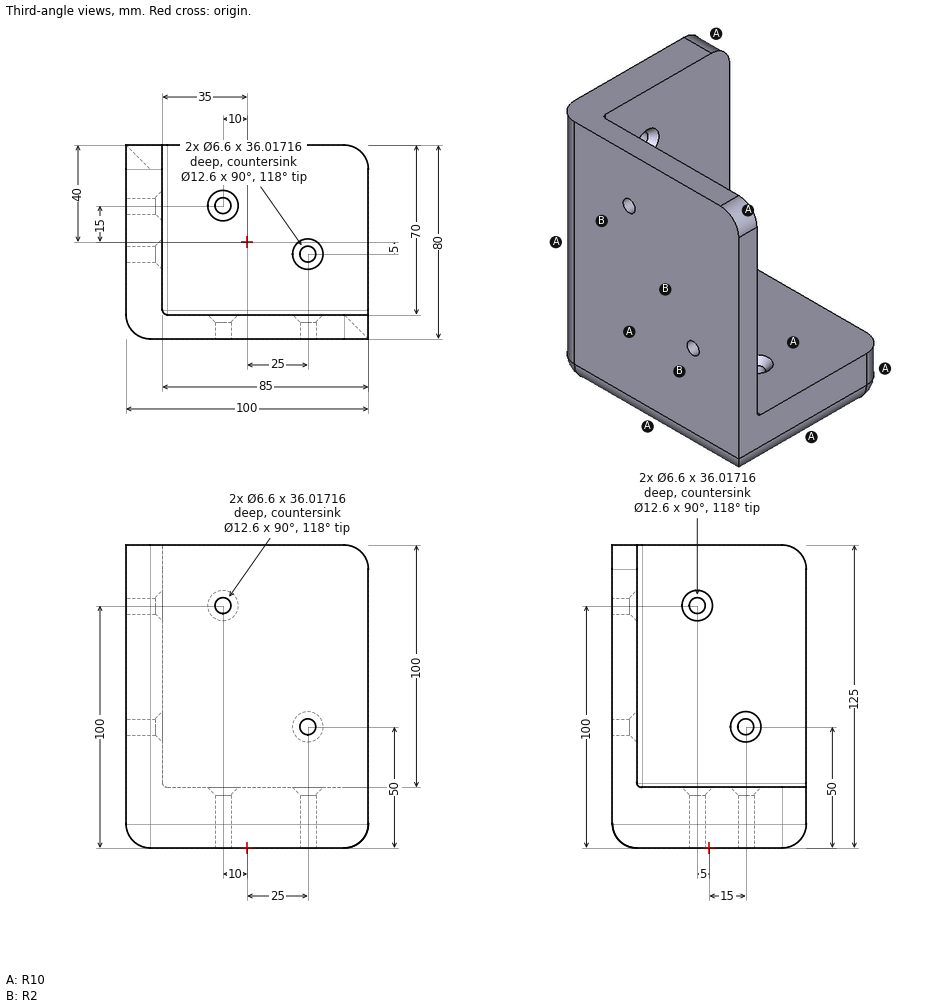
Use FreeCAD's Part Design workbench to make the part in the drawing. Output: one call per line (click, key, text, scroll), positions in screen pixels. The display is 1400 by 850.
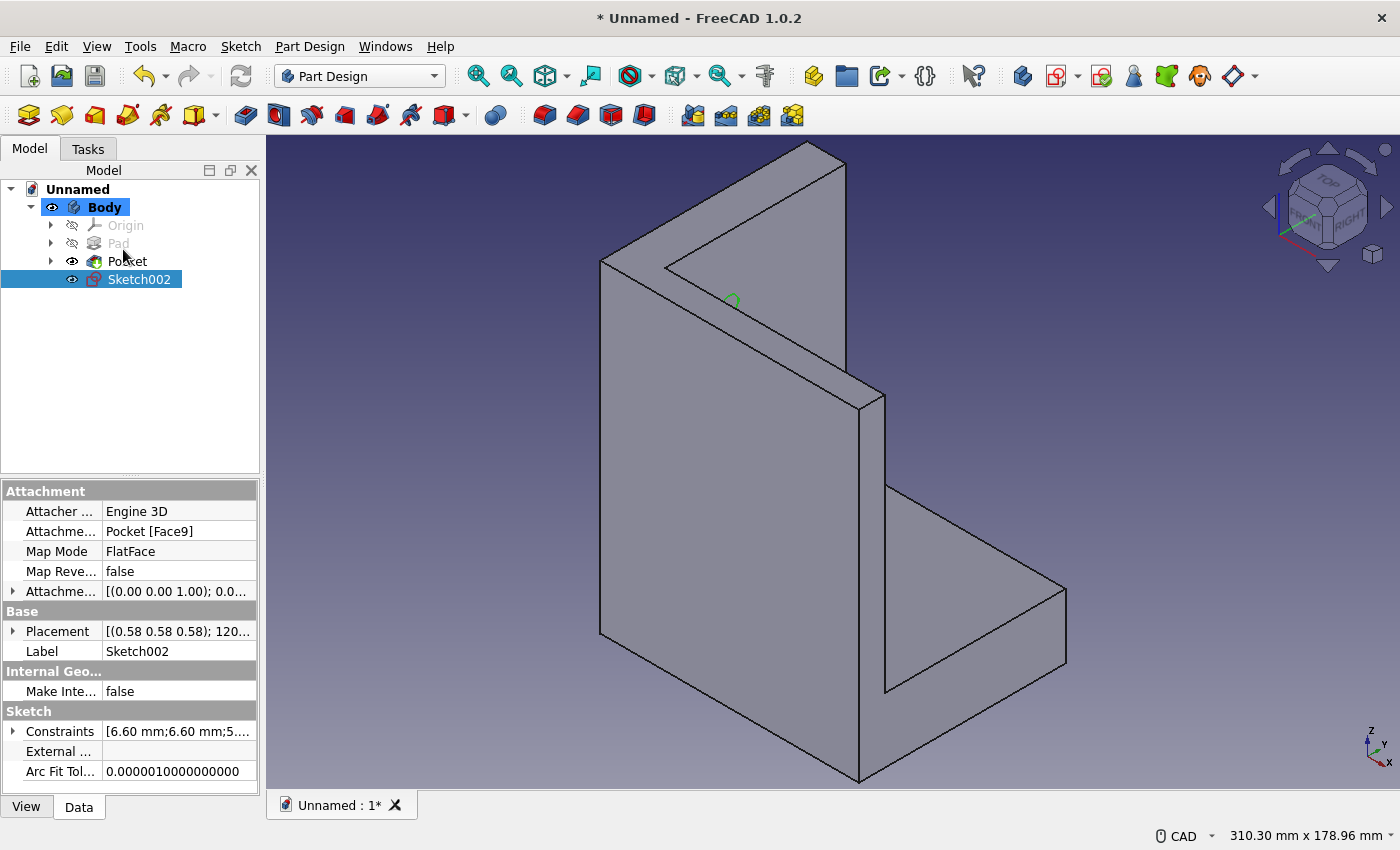
click(279, 116)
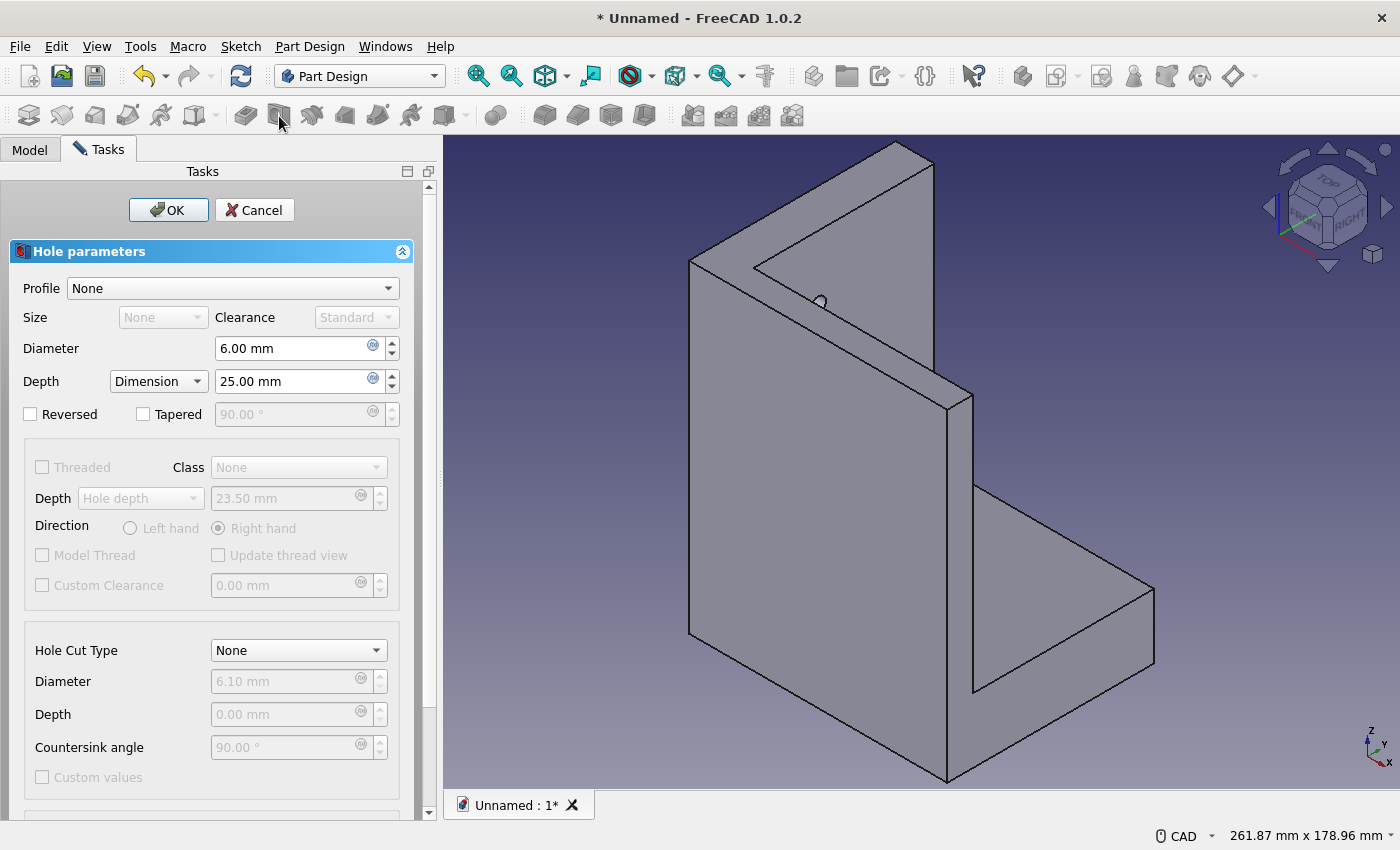
triple_click(300, 348)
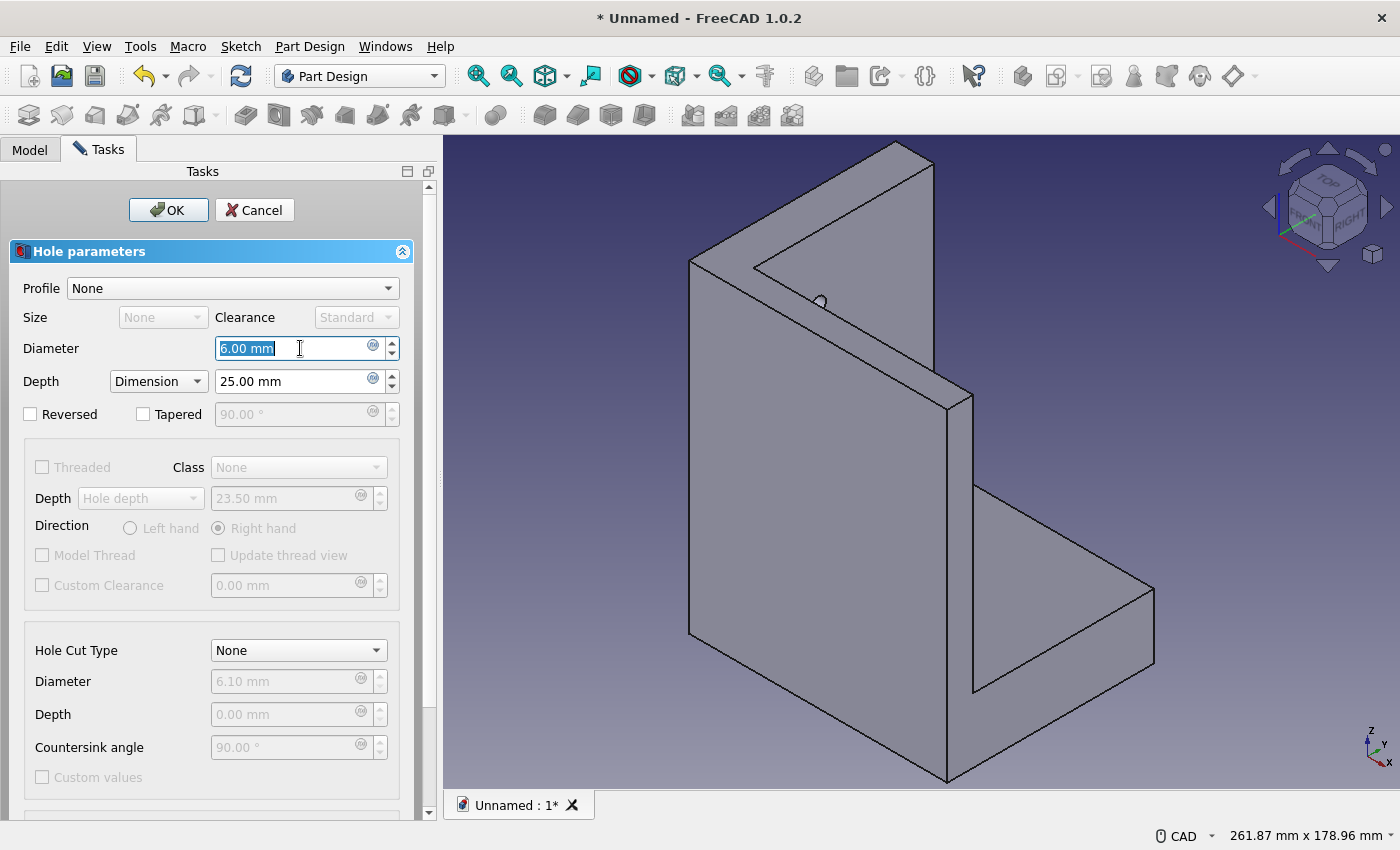
text(6.6)
key(Tab)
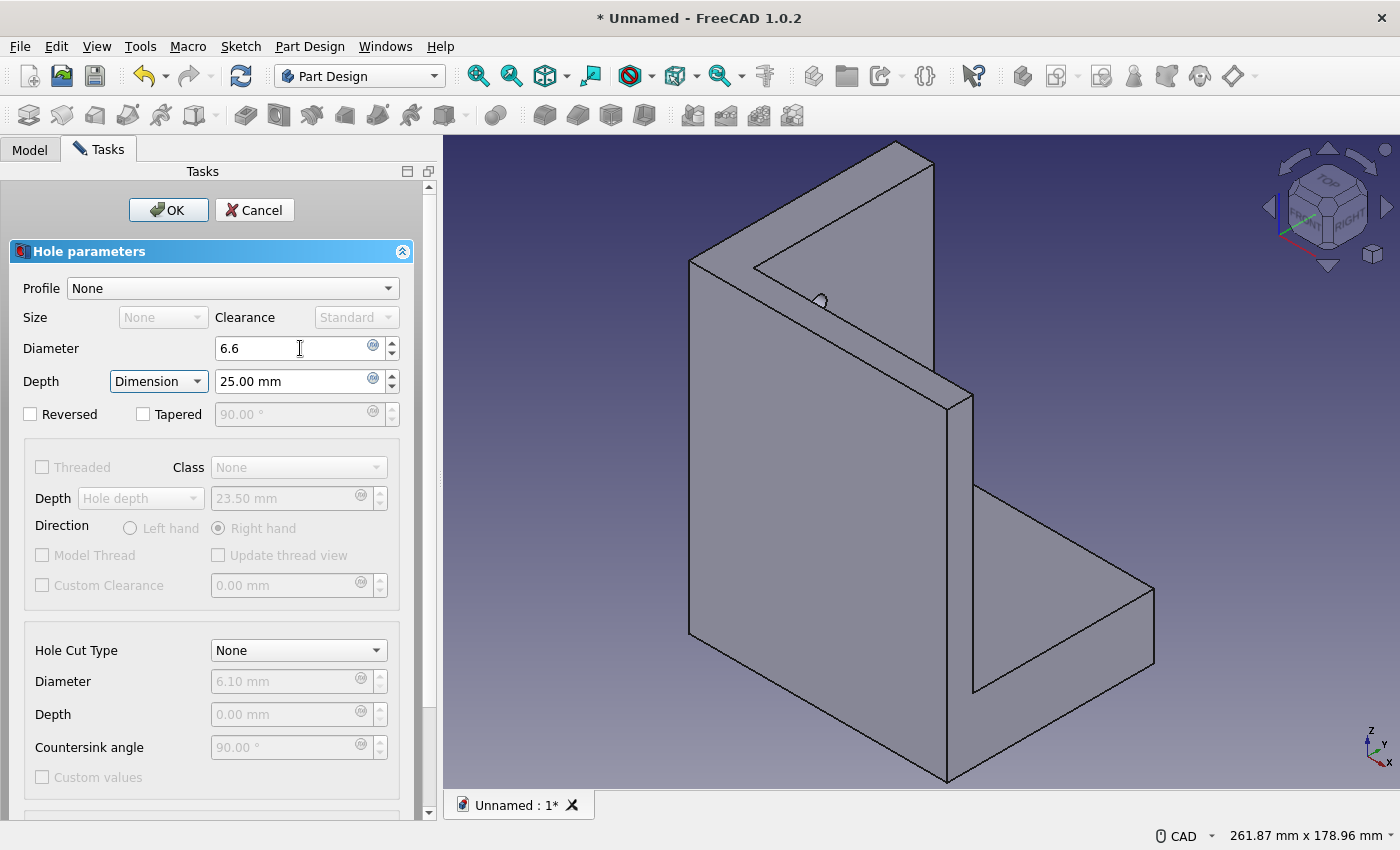
triple_click(300, 382)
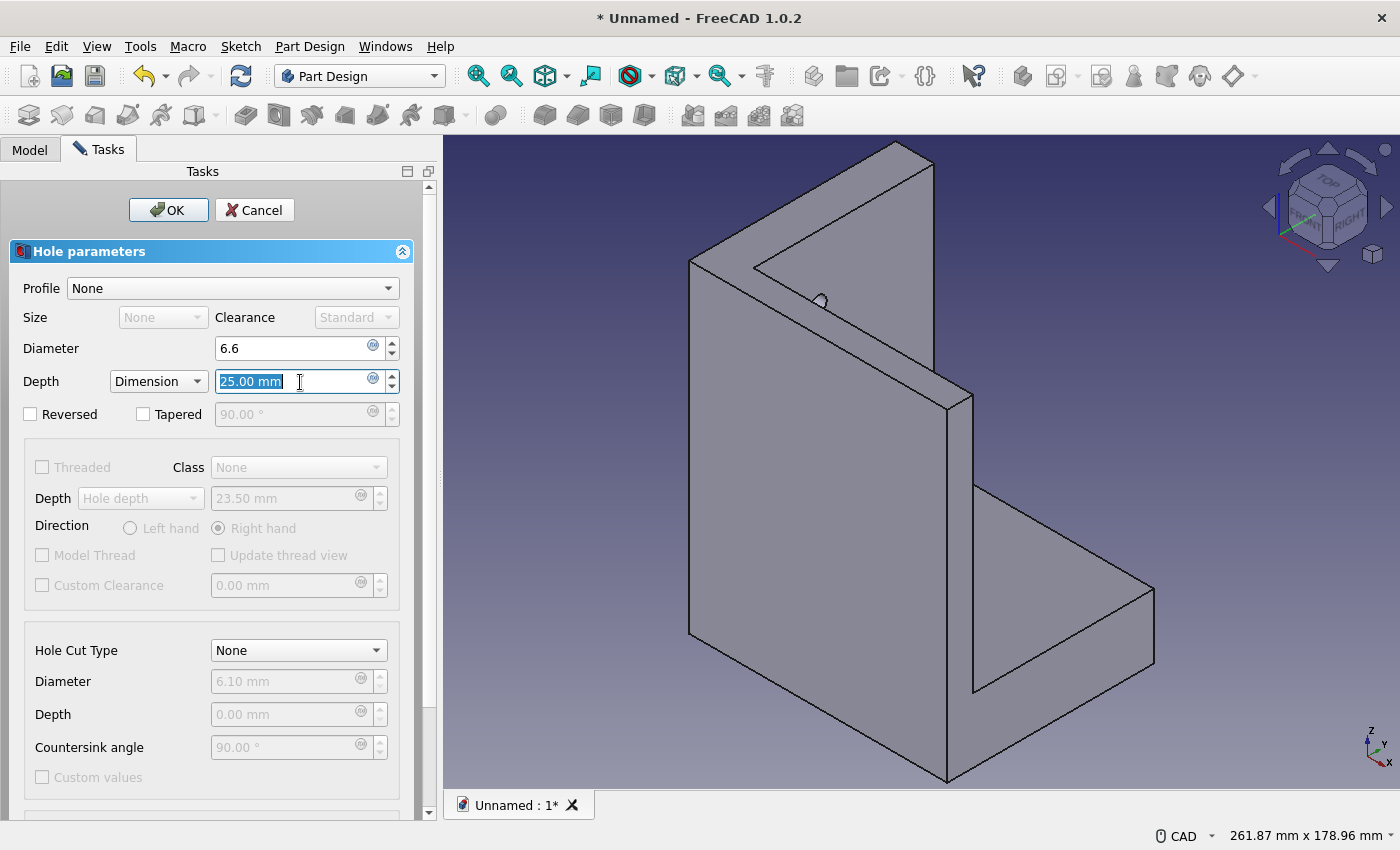
text(36.01716)
key(Tab)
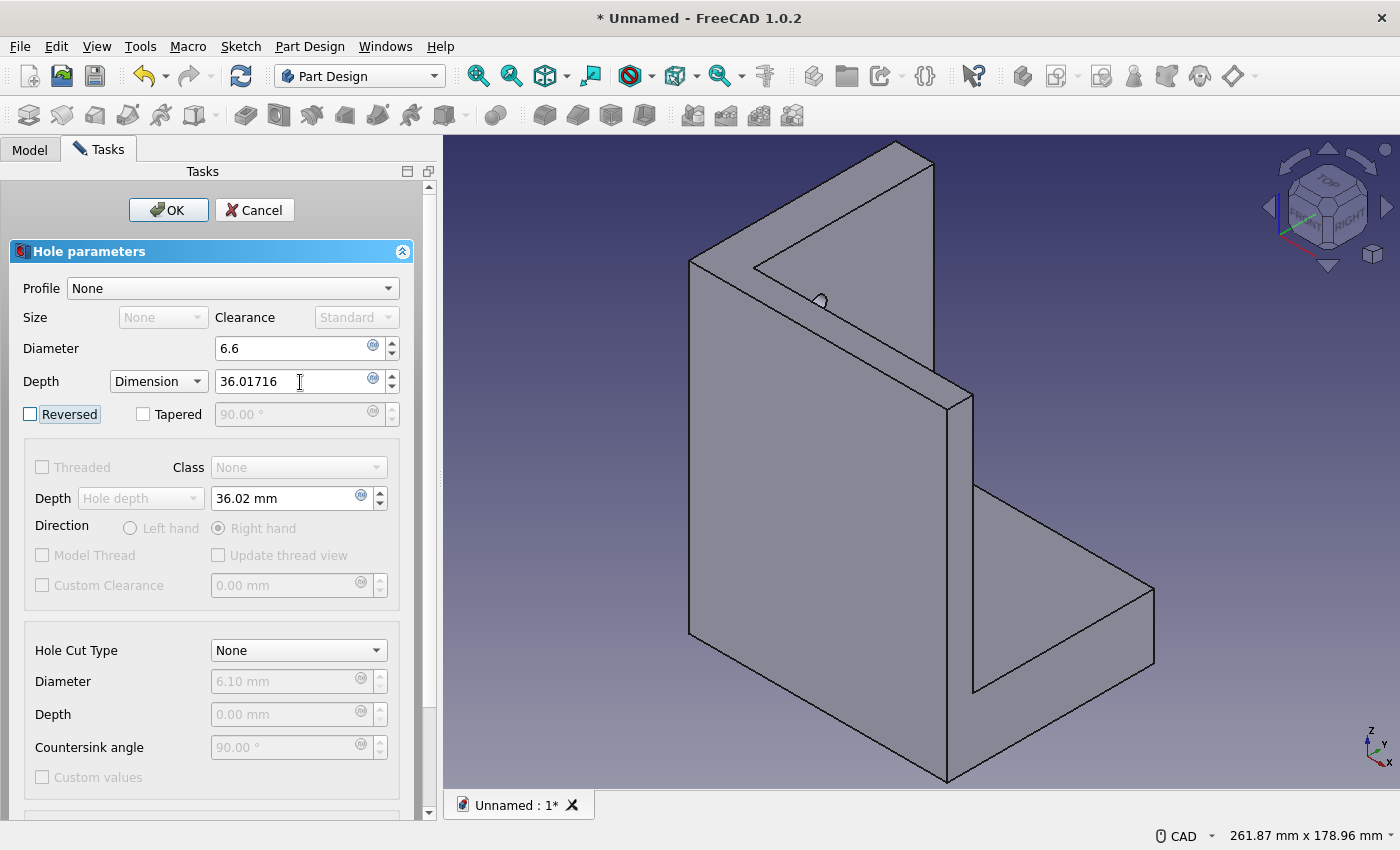
click(300, 650)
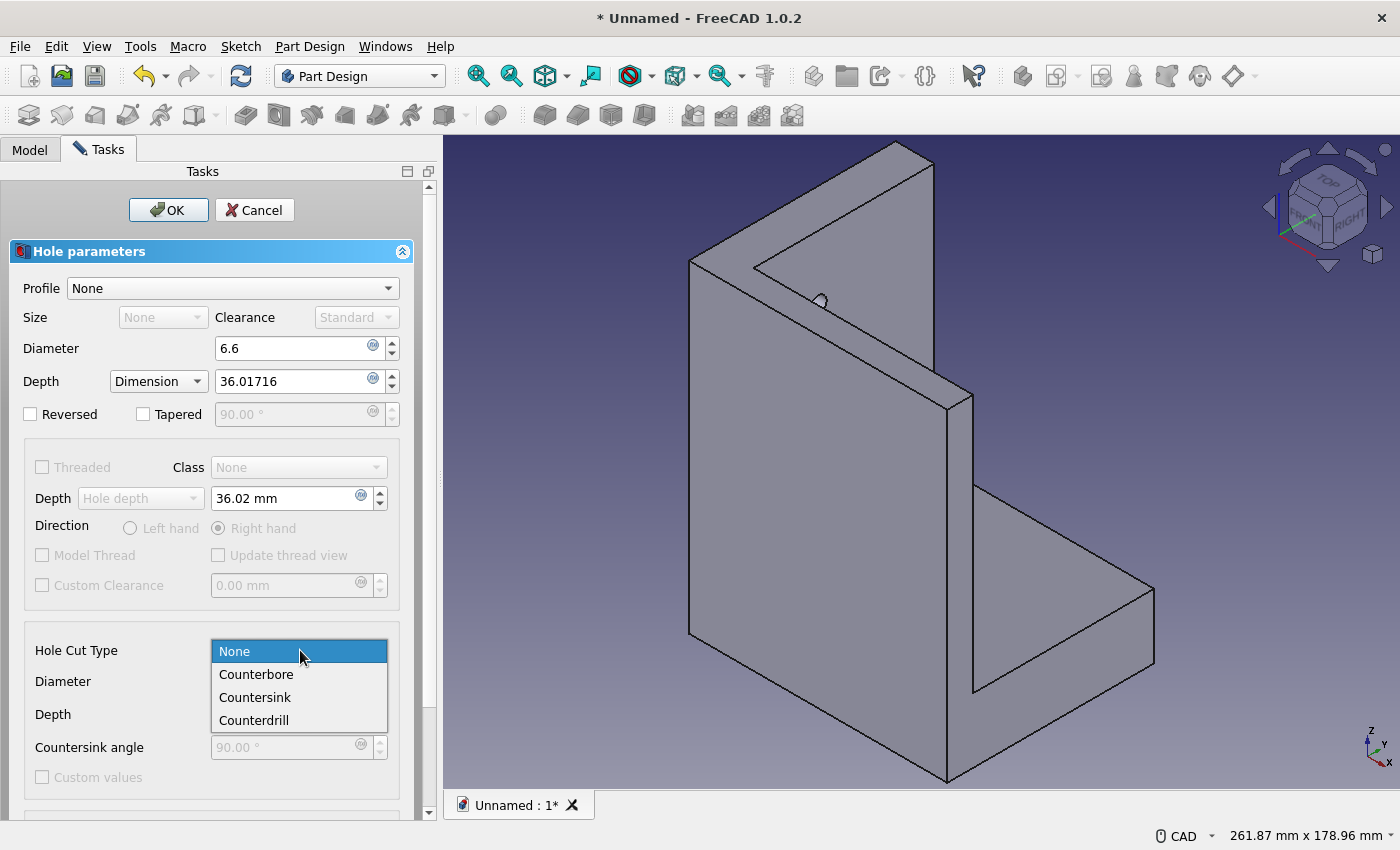
click(298, 698)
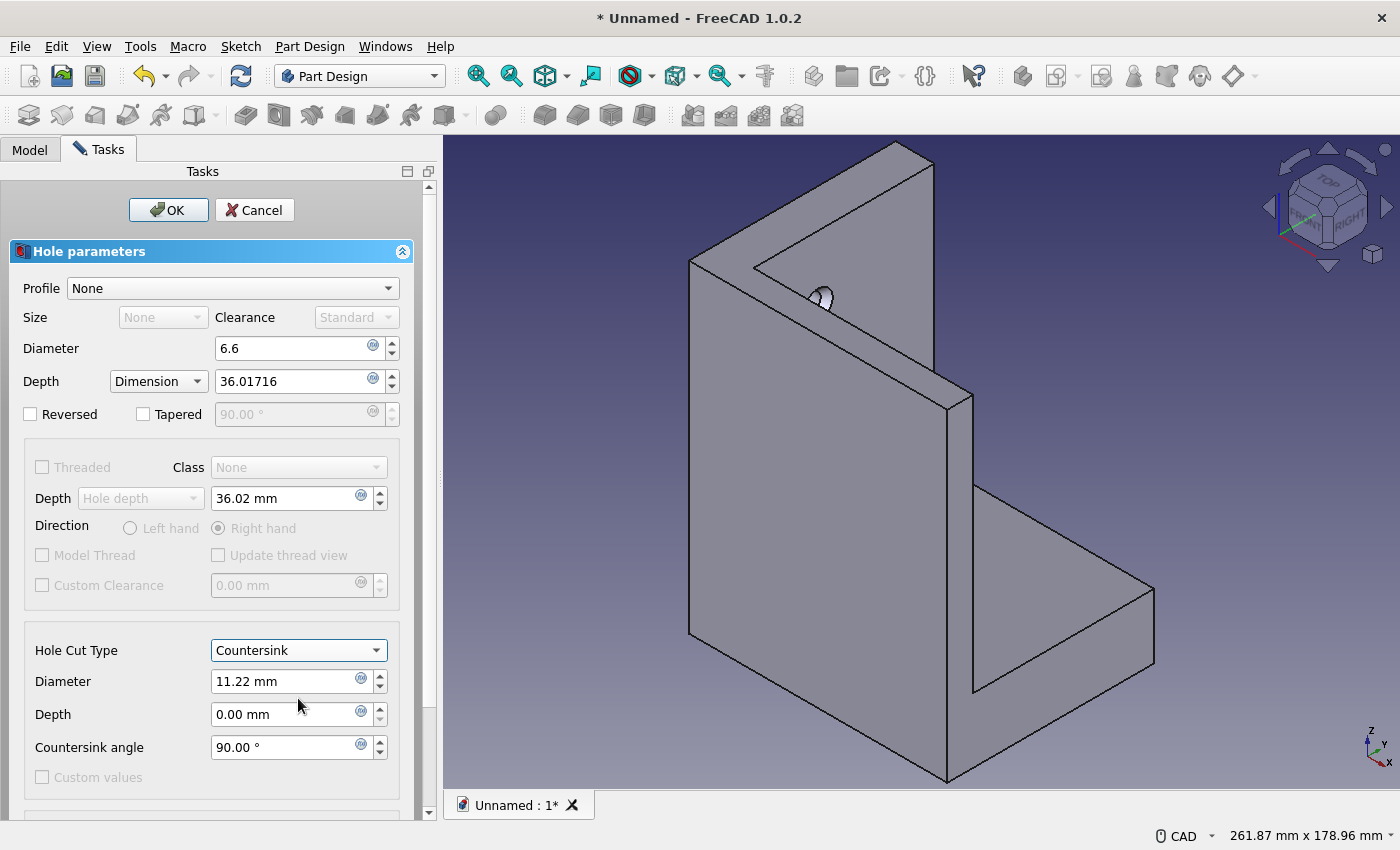
triple_click(292, 682)